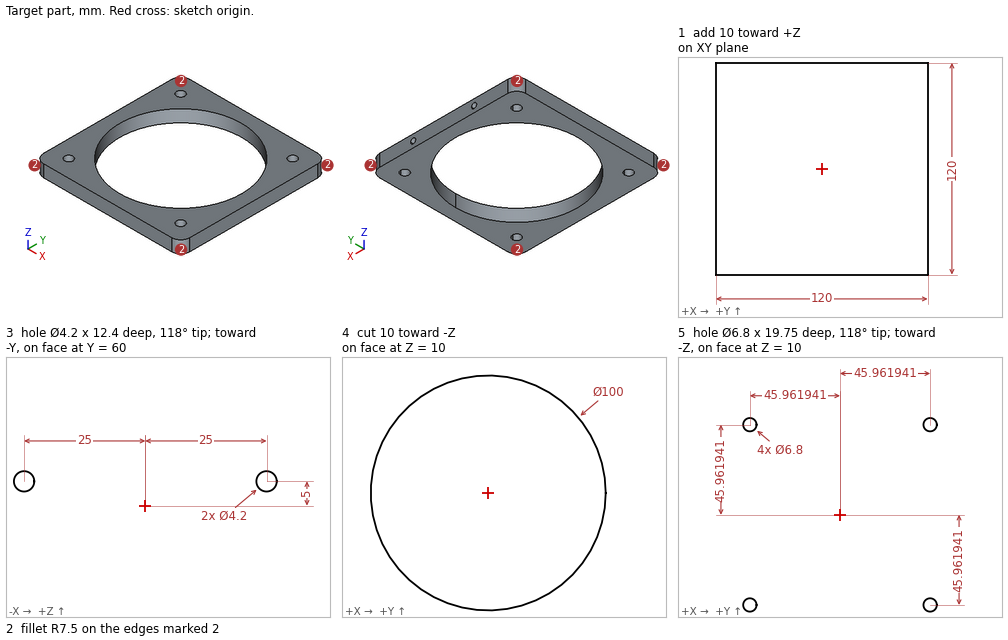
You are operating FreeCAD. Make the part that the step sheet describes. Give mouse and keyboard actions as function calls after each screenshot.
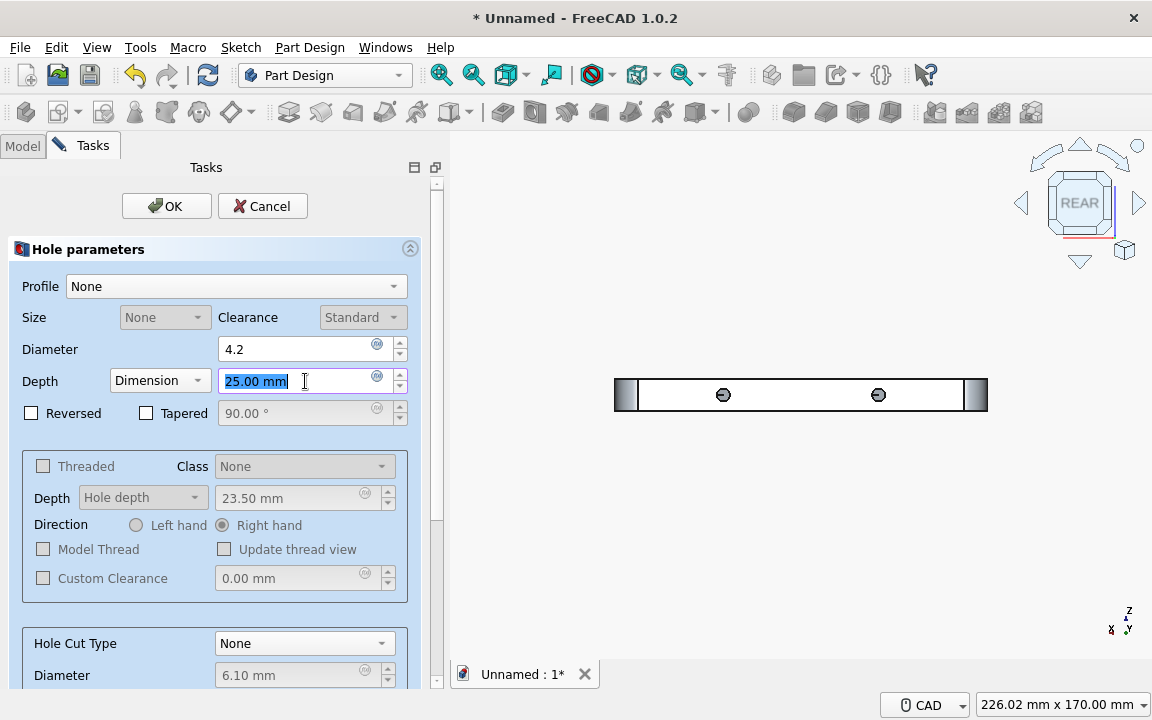
text(12.4)
key(Tab)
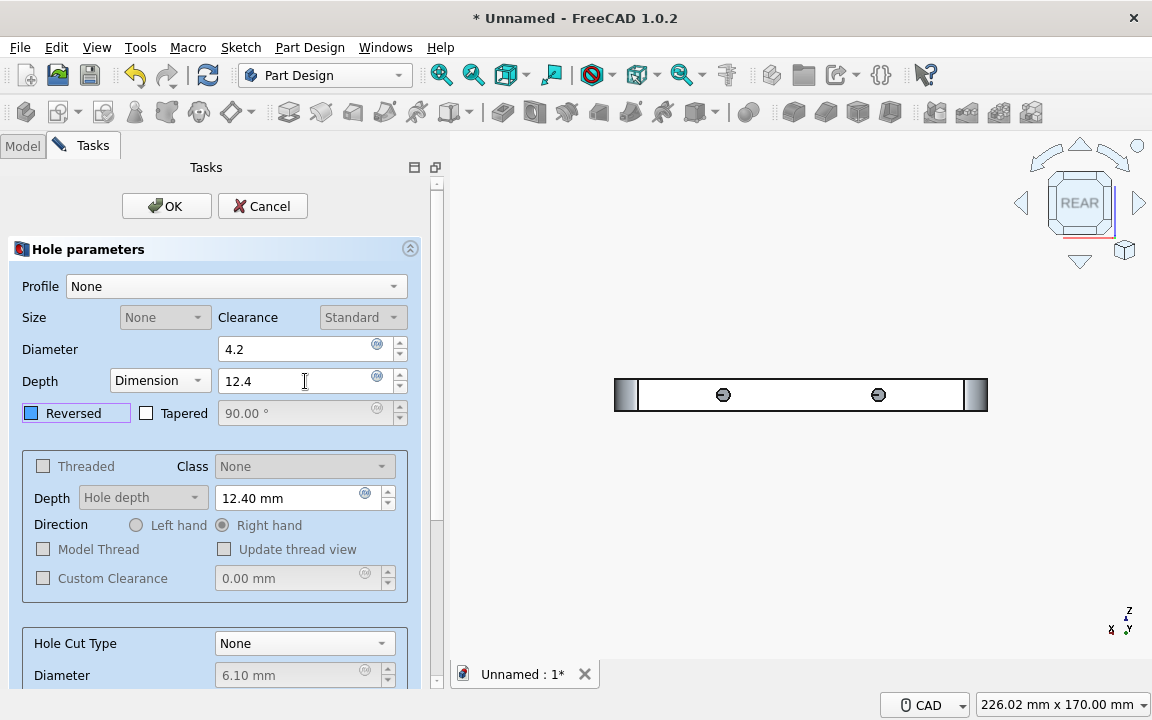
click(167, 206)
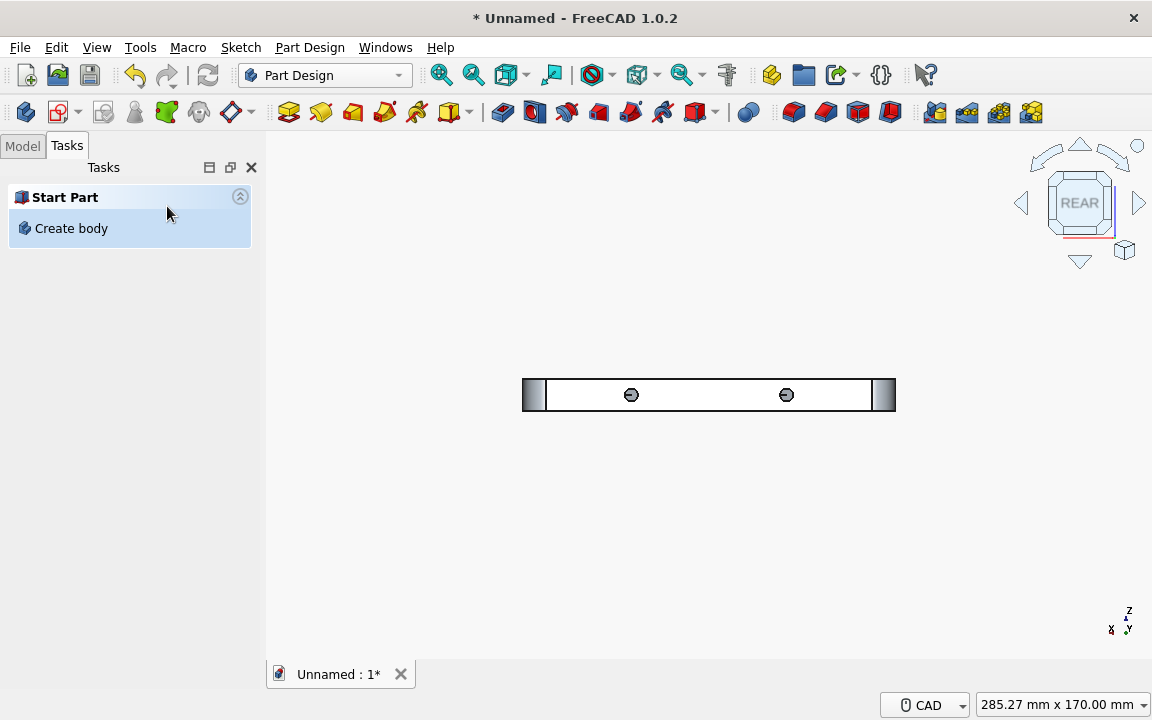
click(442, 76)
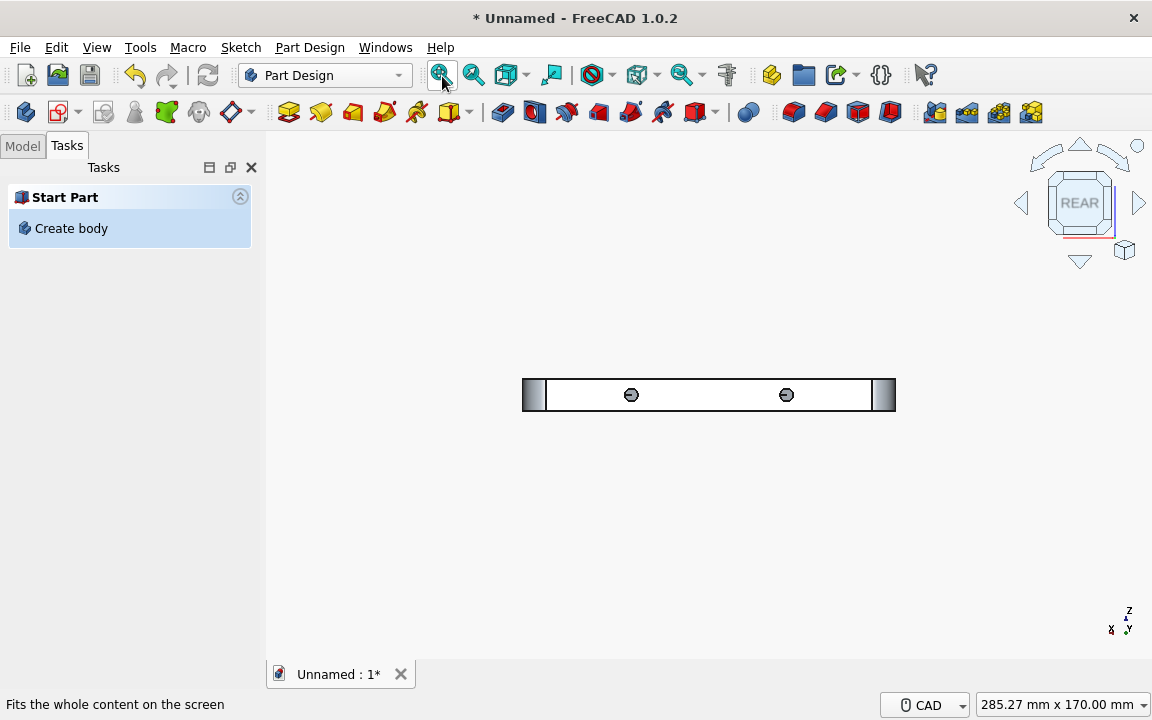
key(0)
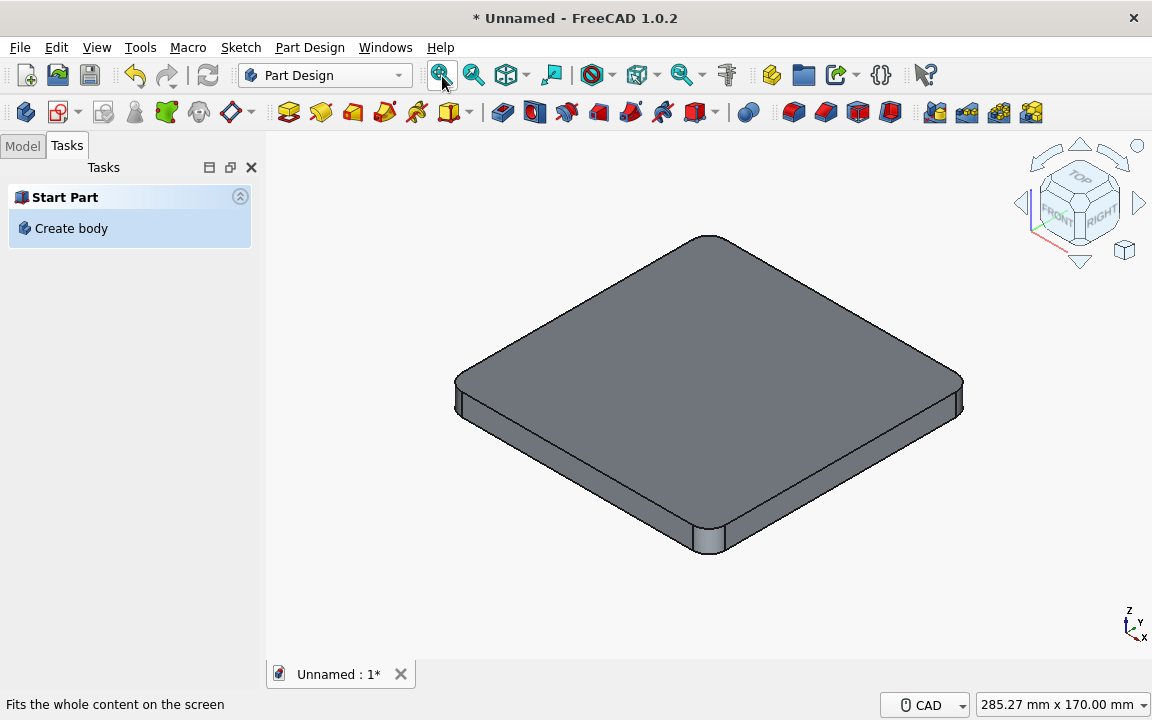
click(709, 381)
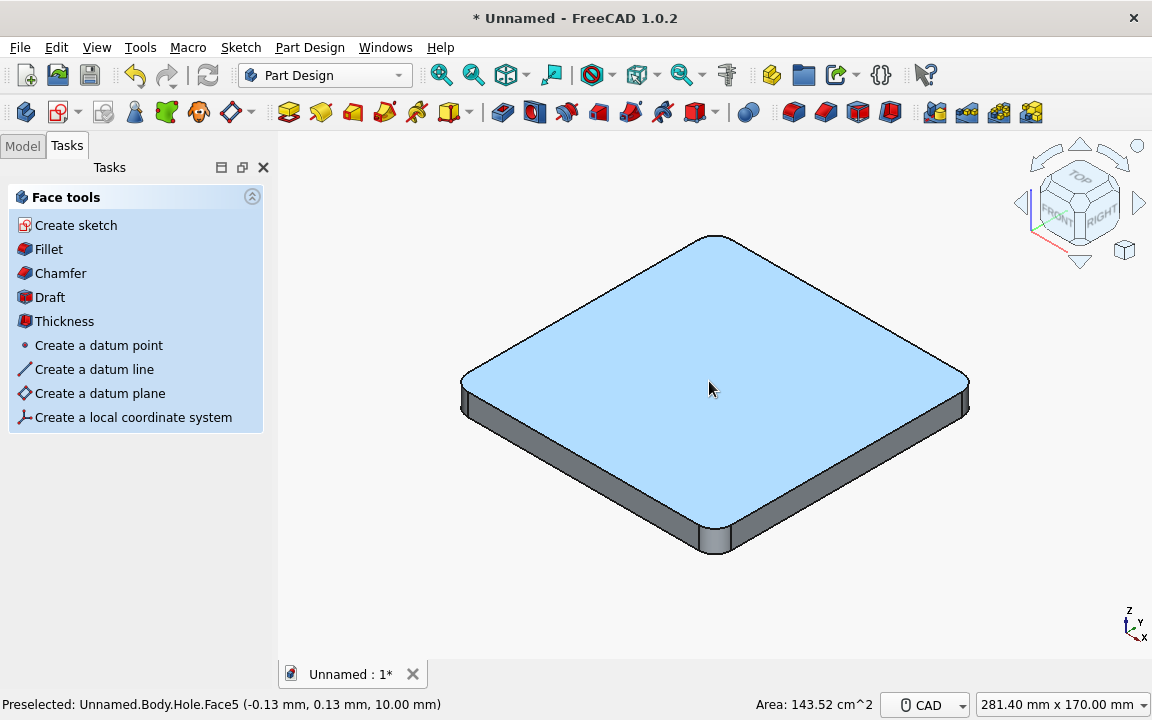
click(58, 112)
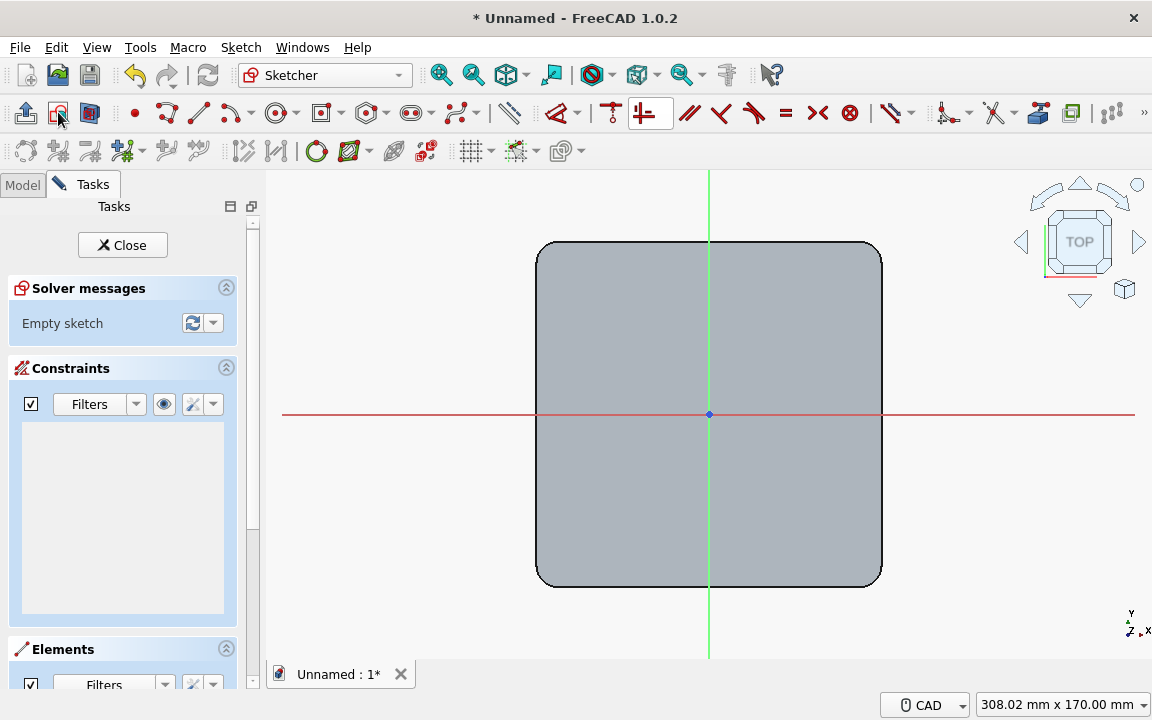
click(276, 114)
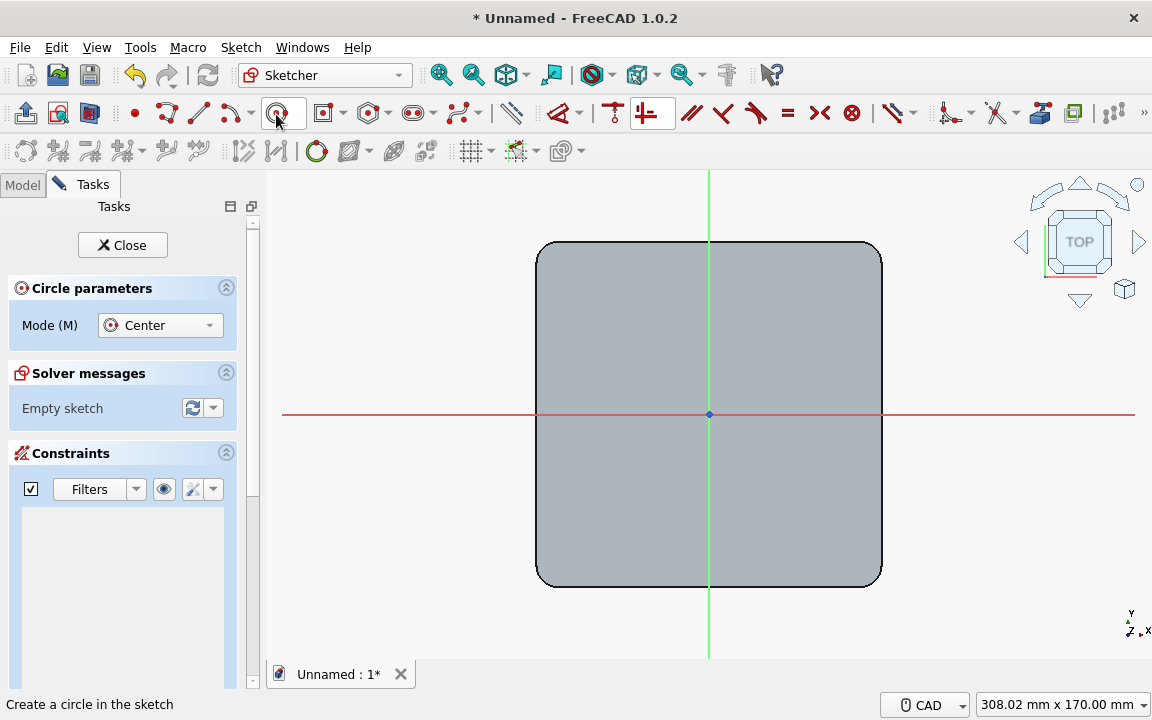
click(709, 415)
click(811, 313)
key(Escape)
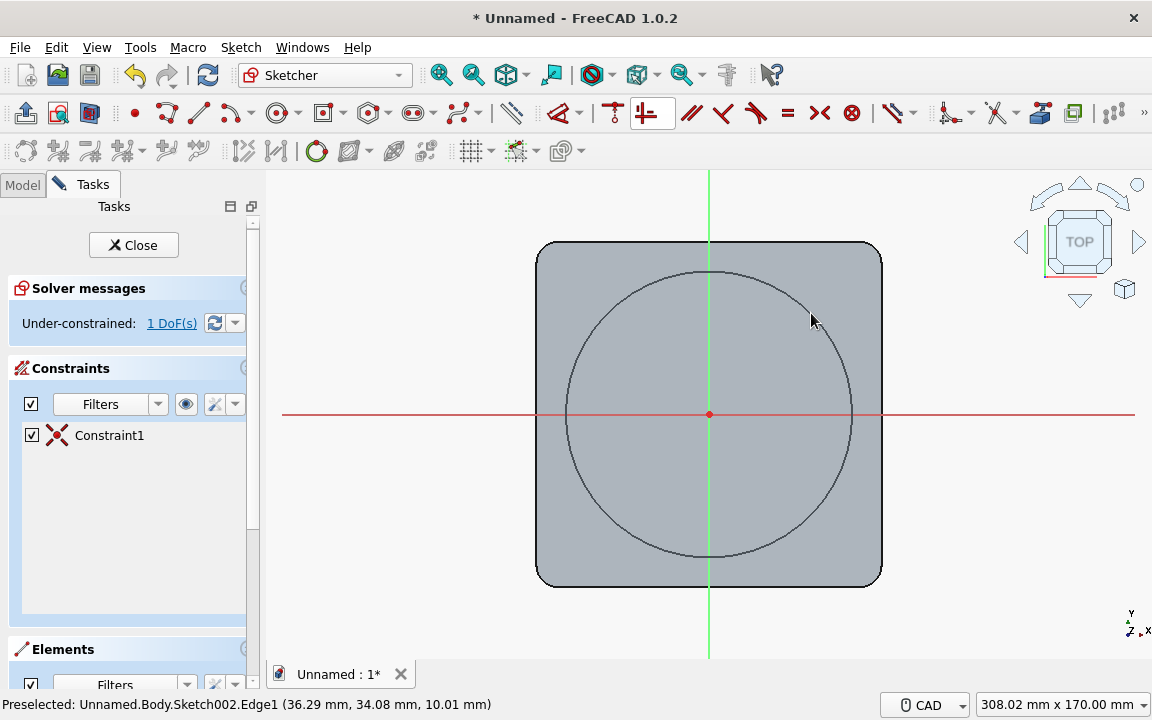
click(558, 114)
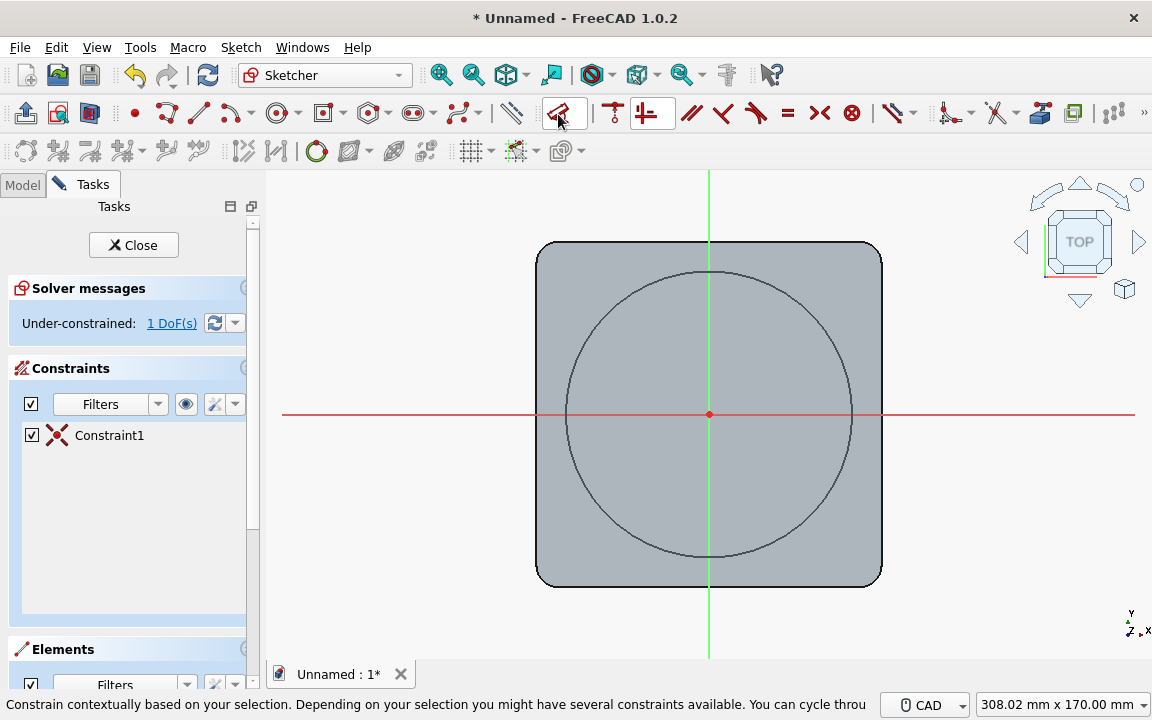
click(810, 313)
click(833, 290)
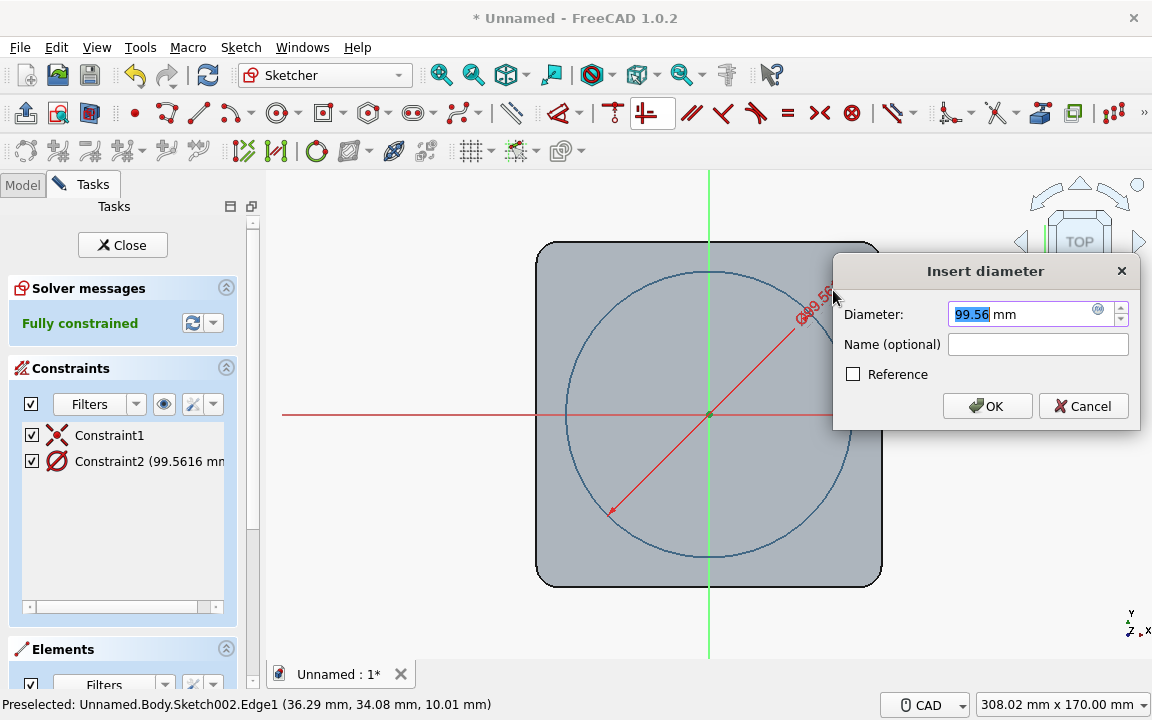
text(100)
key(Return)
key(Escape)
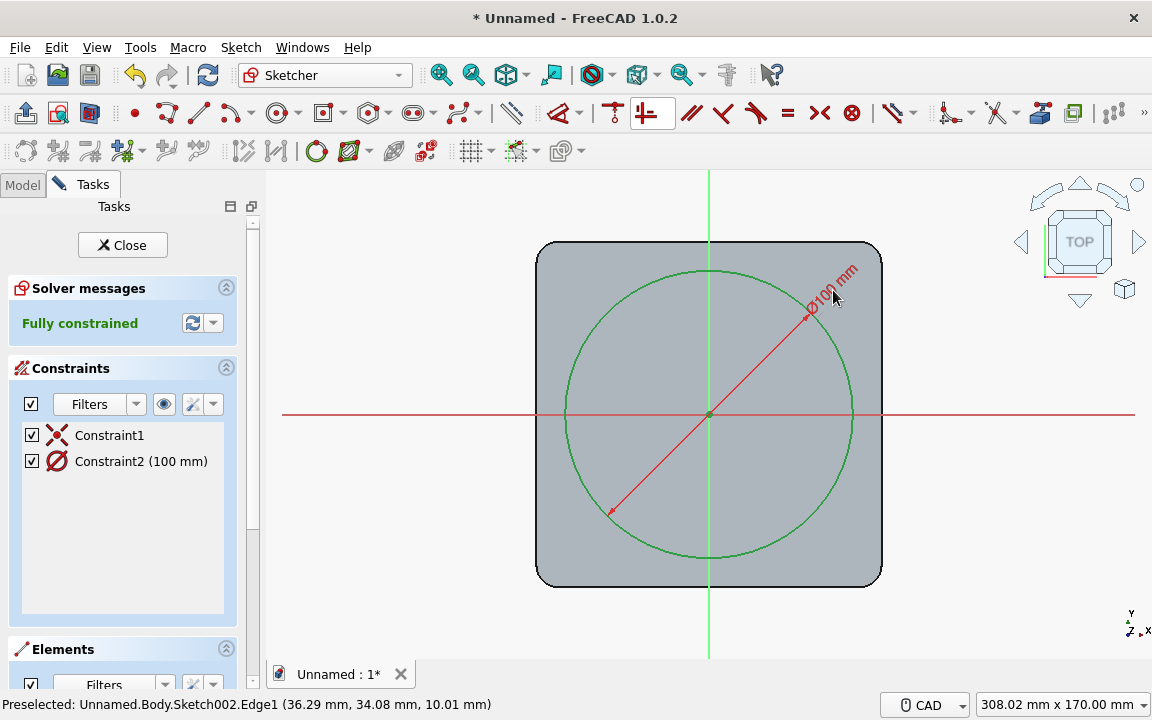
click(123, 245)